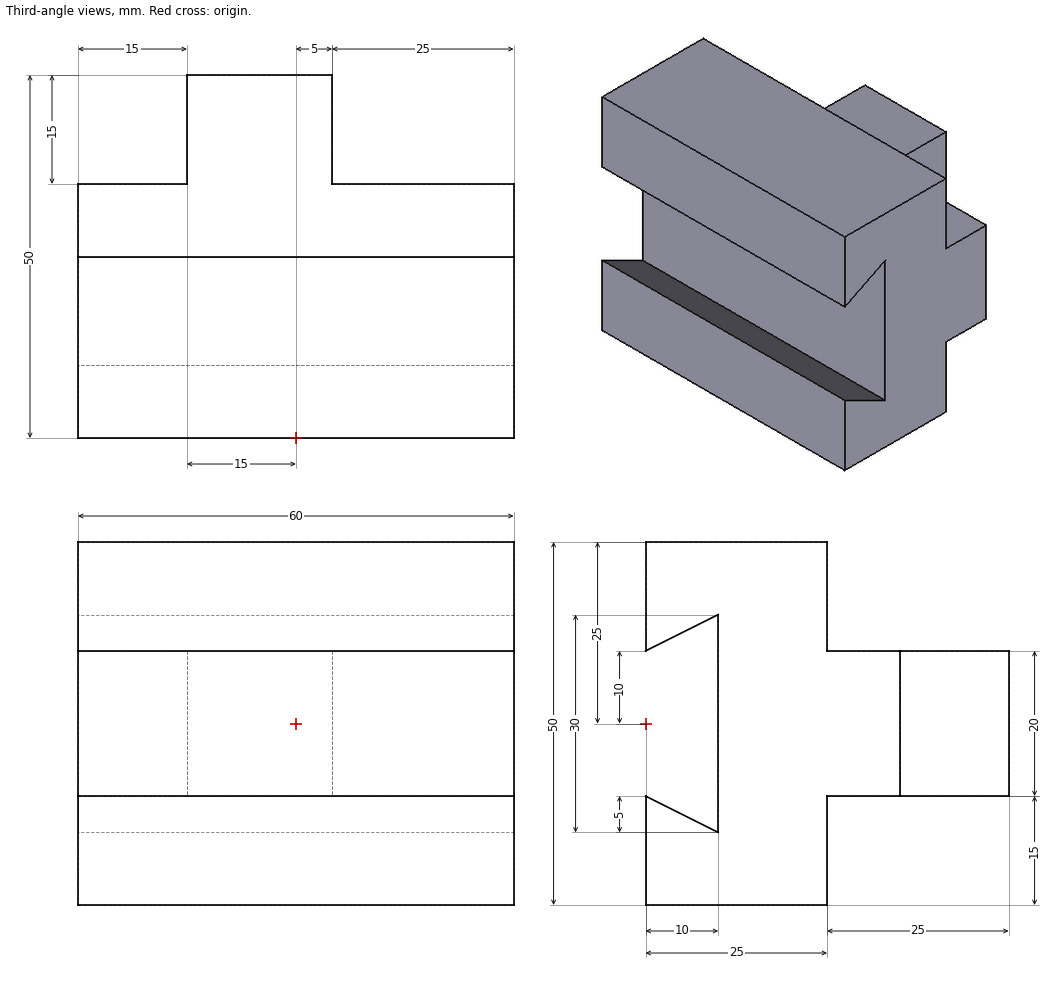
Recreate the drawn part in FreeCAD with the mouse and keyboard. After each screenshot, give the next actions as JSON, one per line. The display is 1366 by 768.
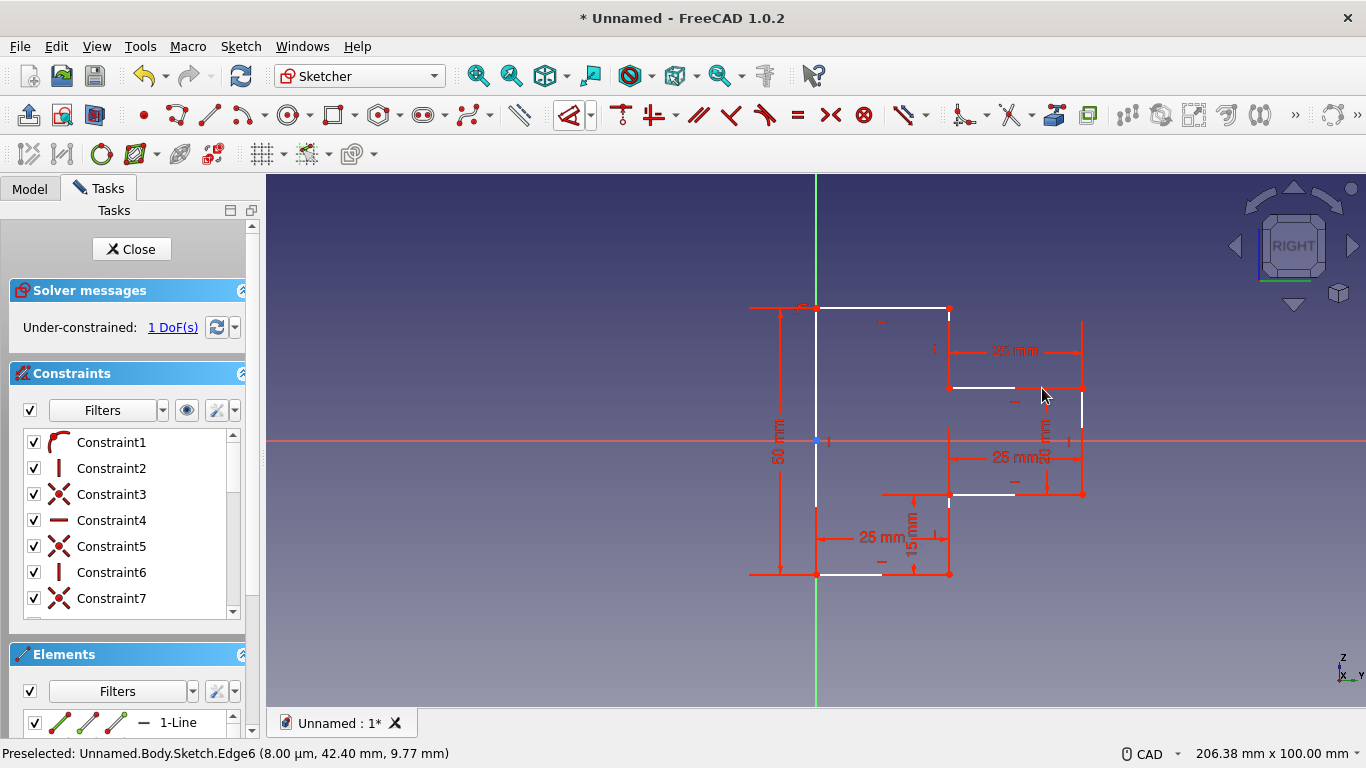
{"action": "left_click", "coordinate": [816, 308]}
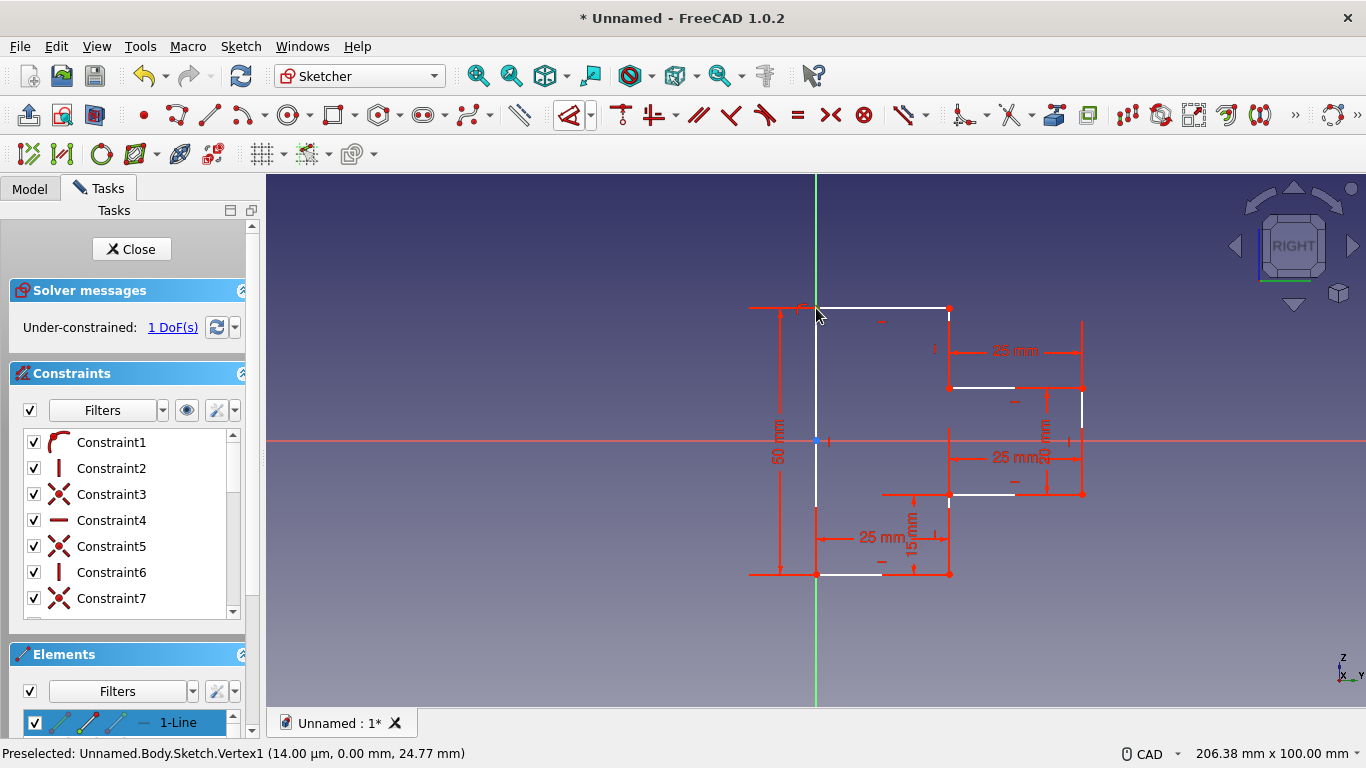
{"action": "key", "text": "i"}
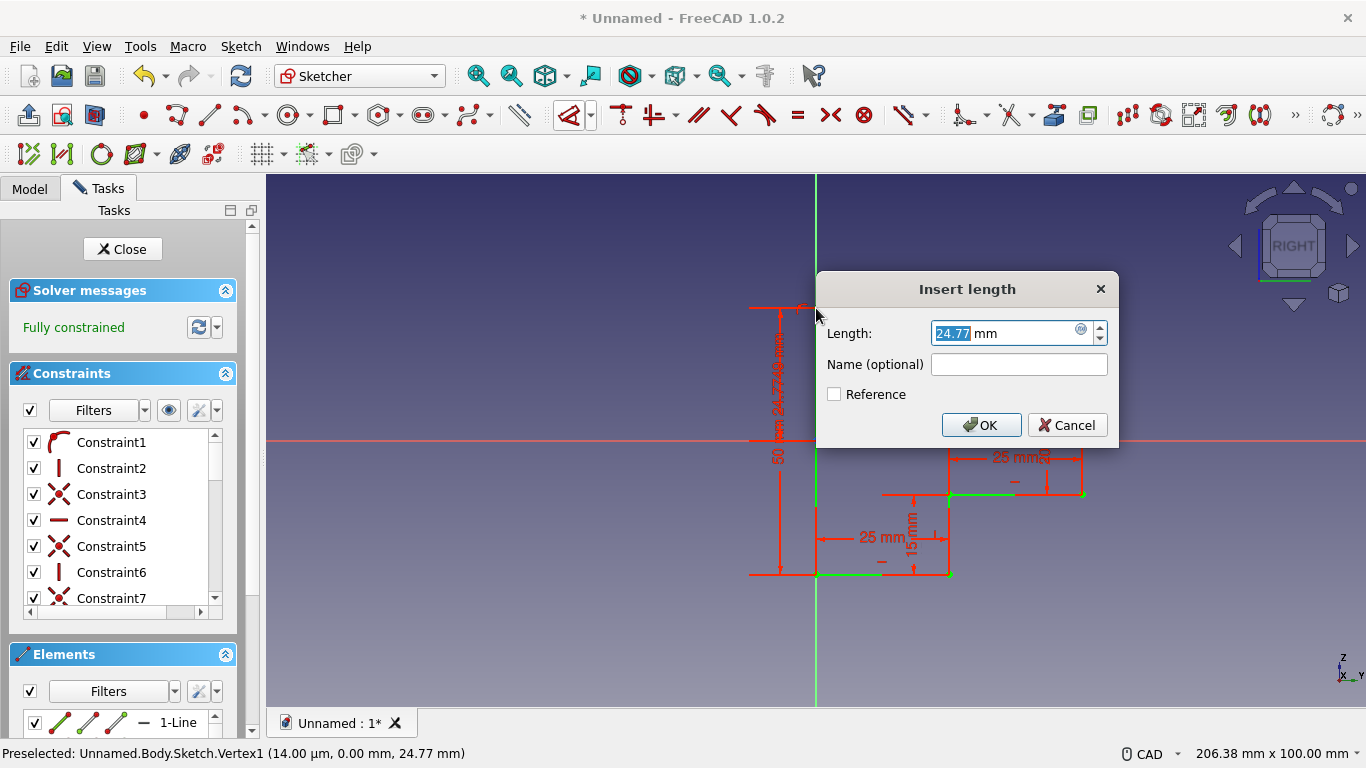
{"action": "type", "text": "25"}
{"action": "key", "text": "Return"}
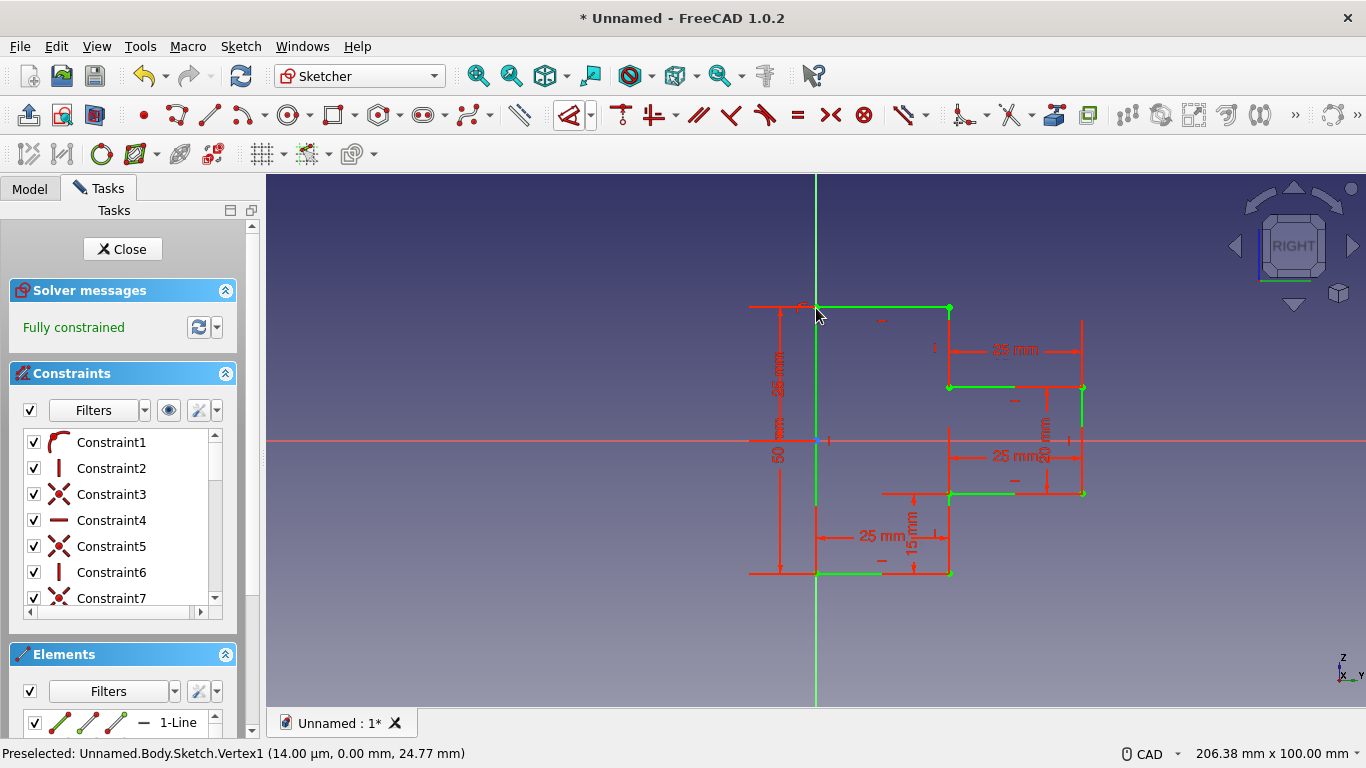
{"action": "left_click", "coordinate": [123, 249]}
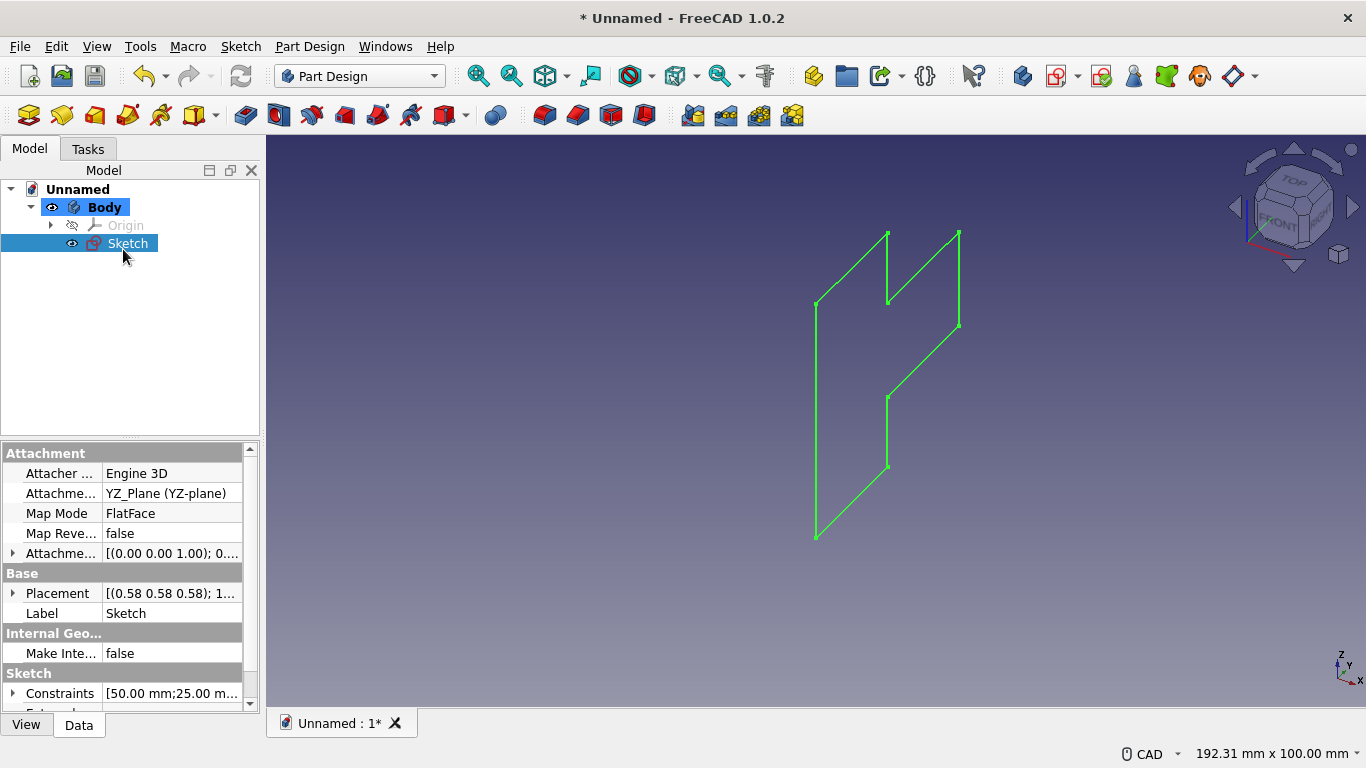
{"action": "left_click", "coordinate": [29, 116]}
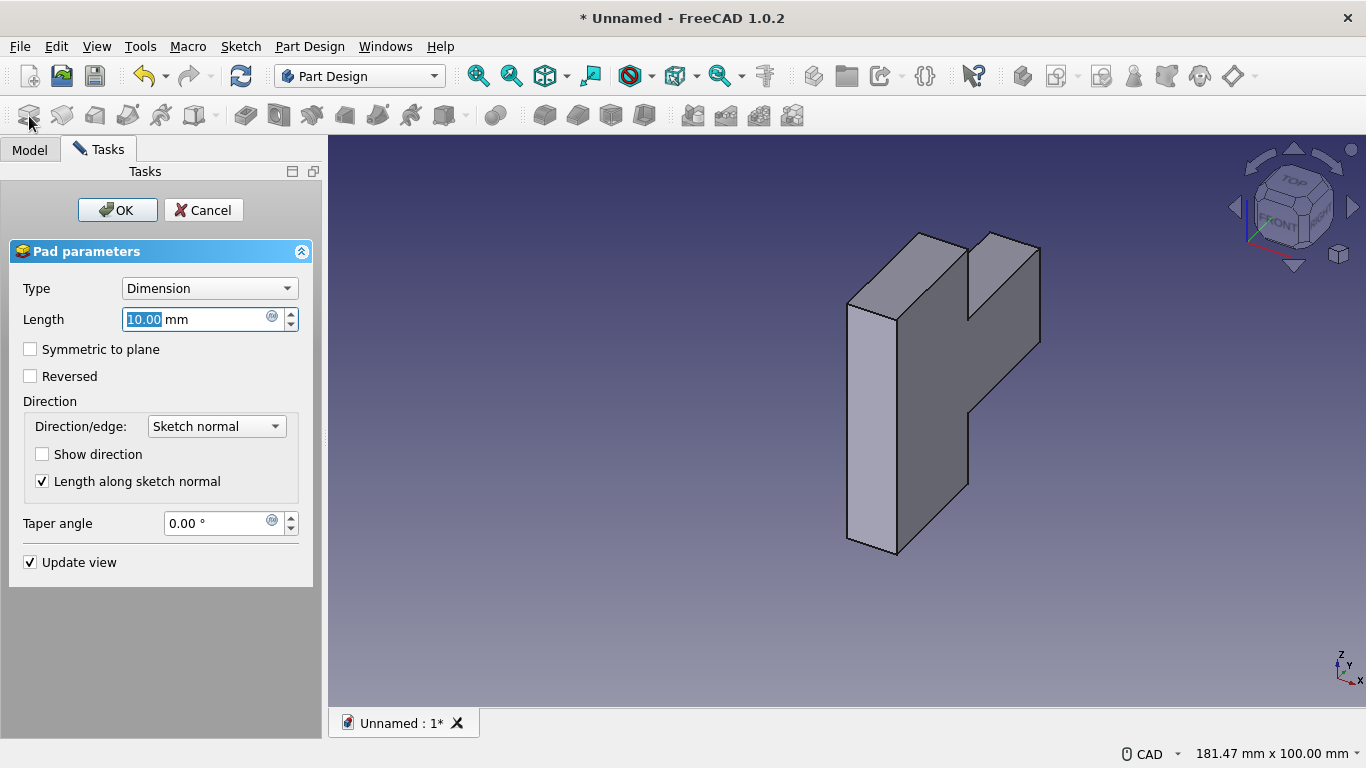
{"action": "type", "text": "60"}
{"action": "key", "text": "Tab"}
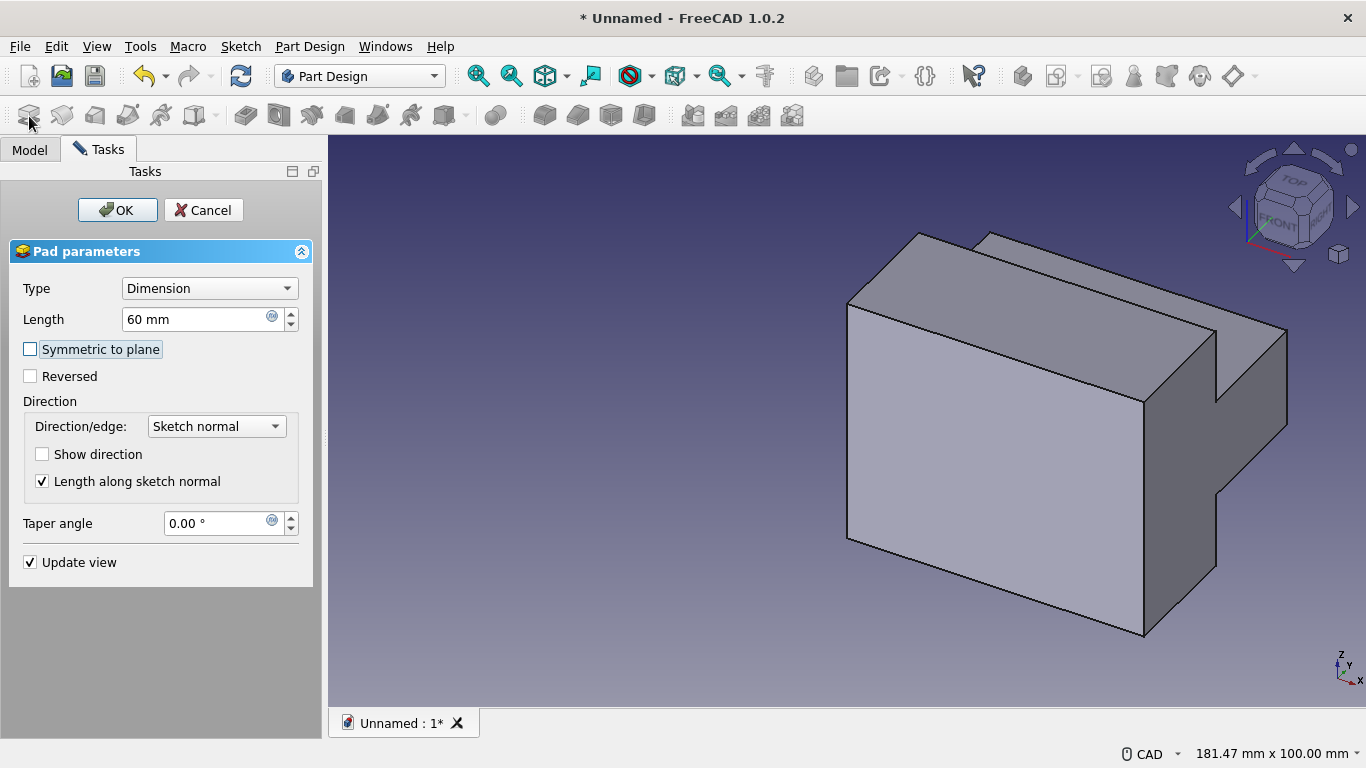
{"action": "left_click", "coordinate": [31, 349]}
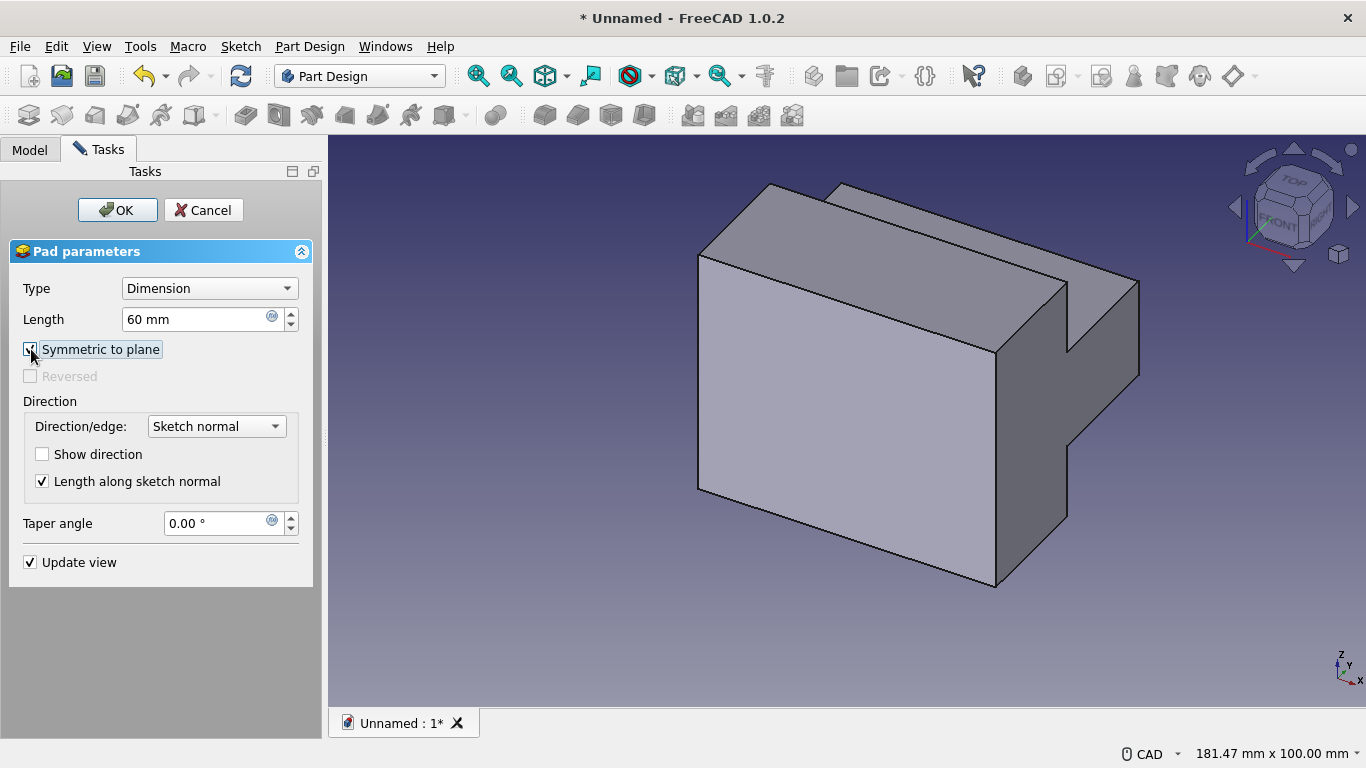
{"action": "left_click", "coordinate": [118, 210]}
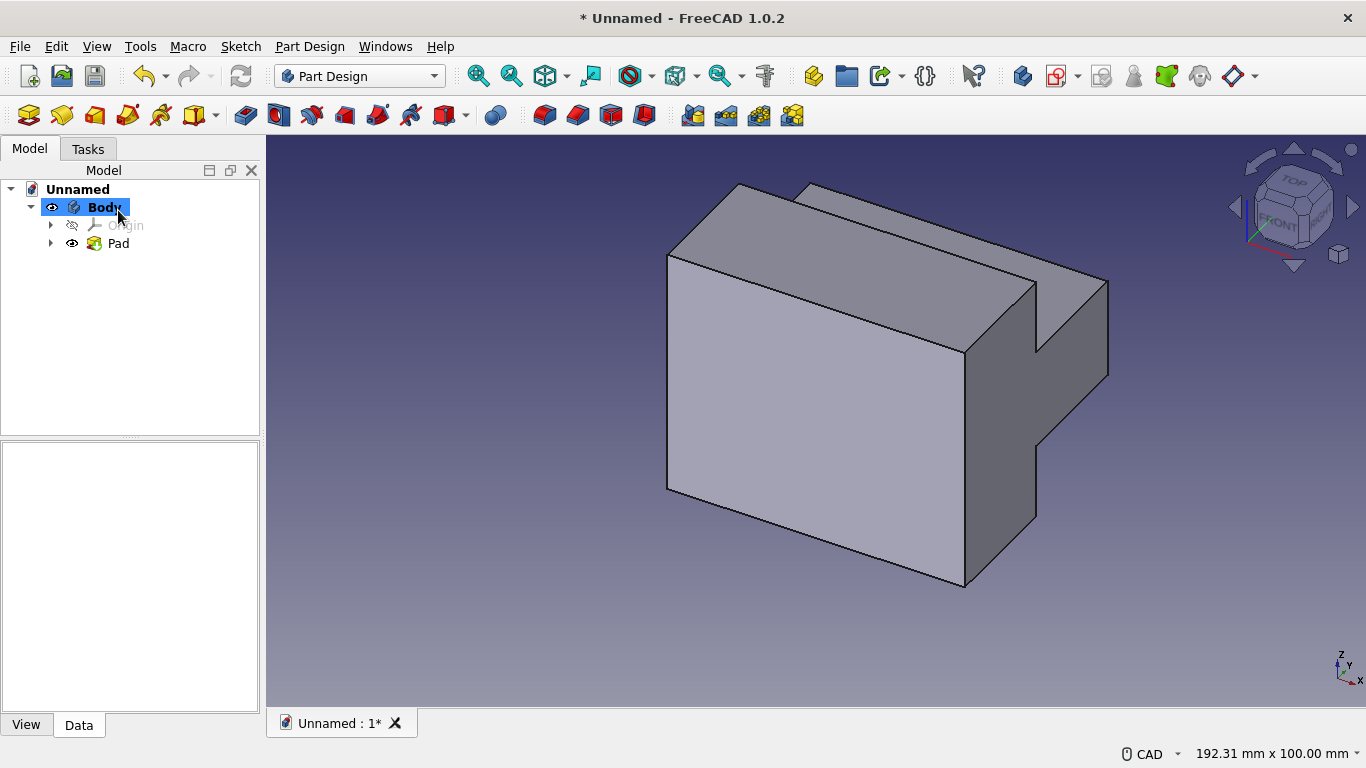
{"action": "key", "text": "v f"}